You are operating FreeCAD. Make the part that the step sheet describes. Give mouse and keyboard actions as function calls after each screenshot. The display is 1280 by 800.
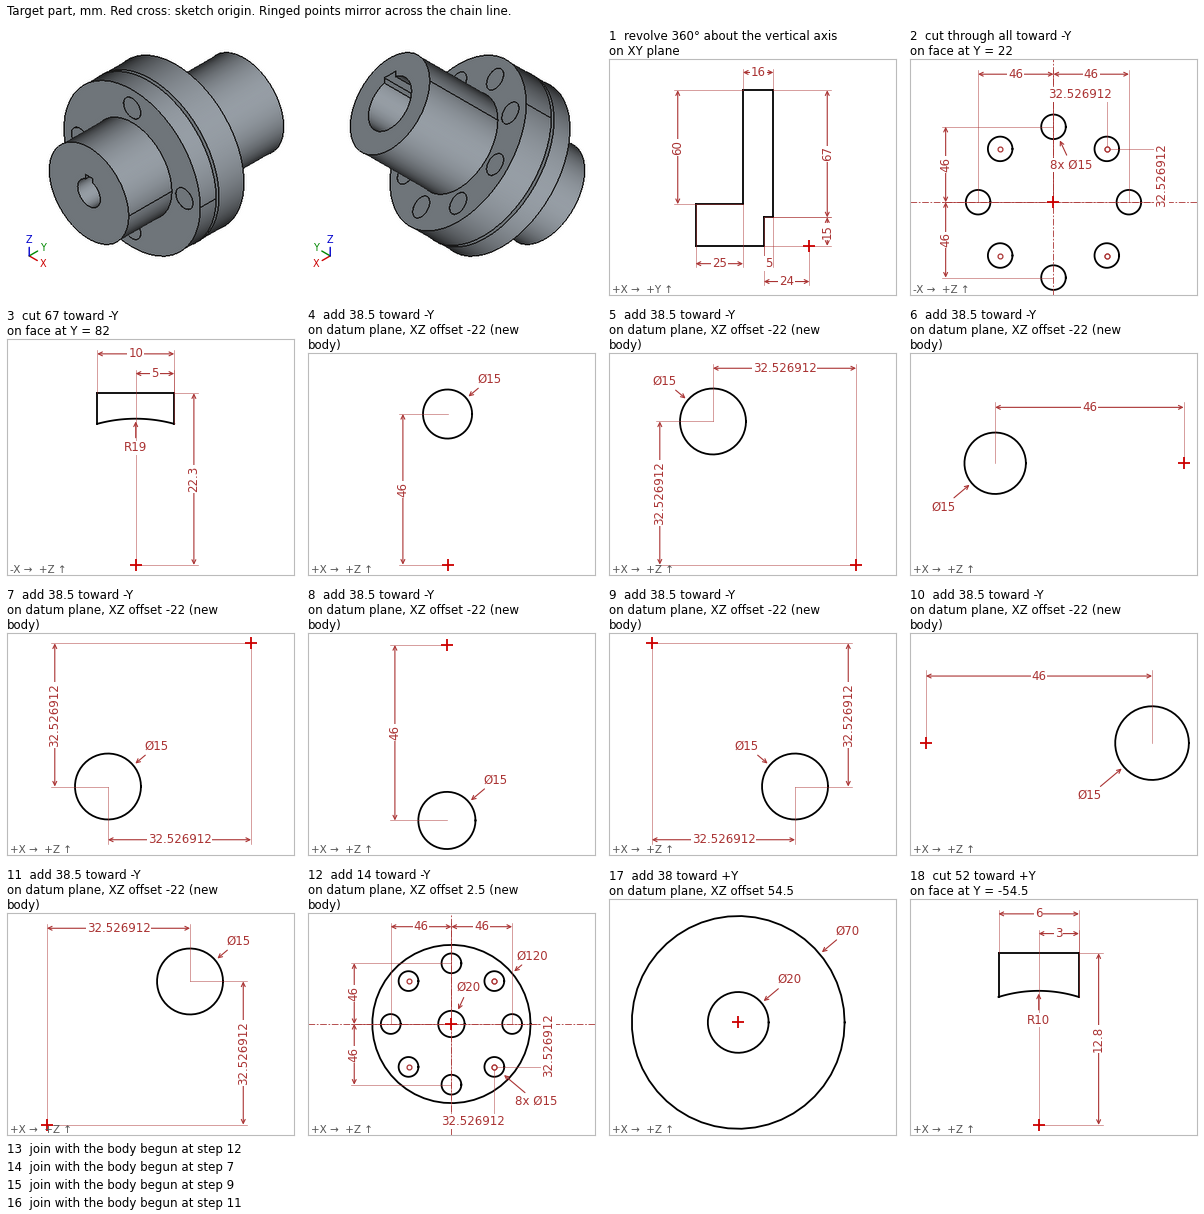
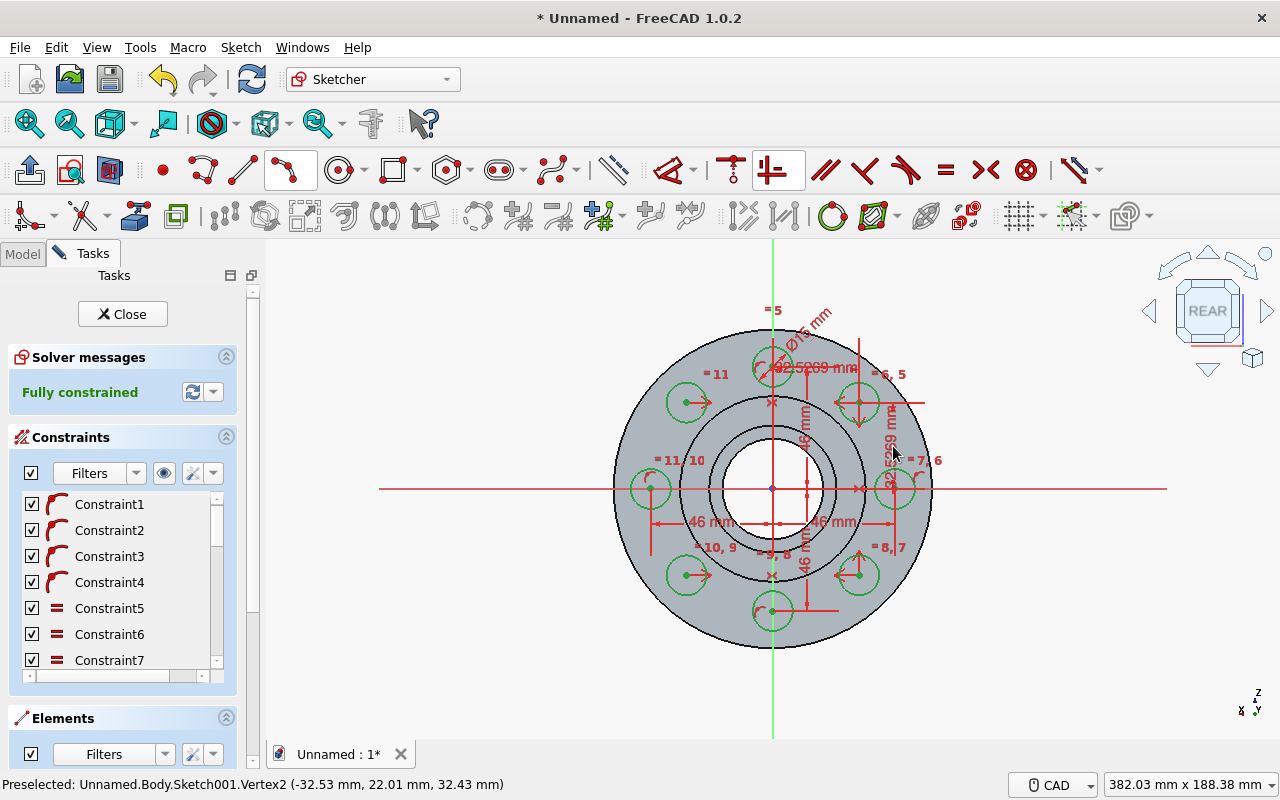
click(123, 314)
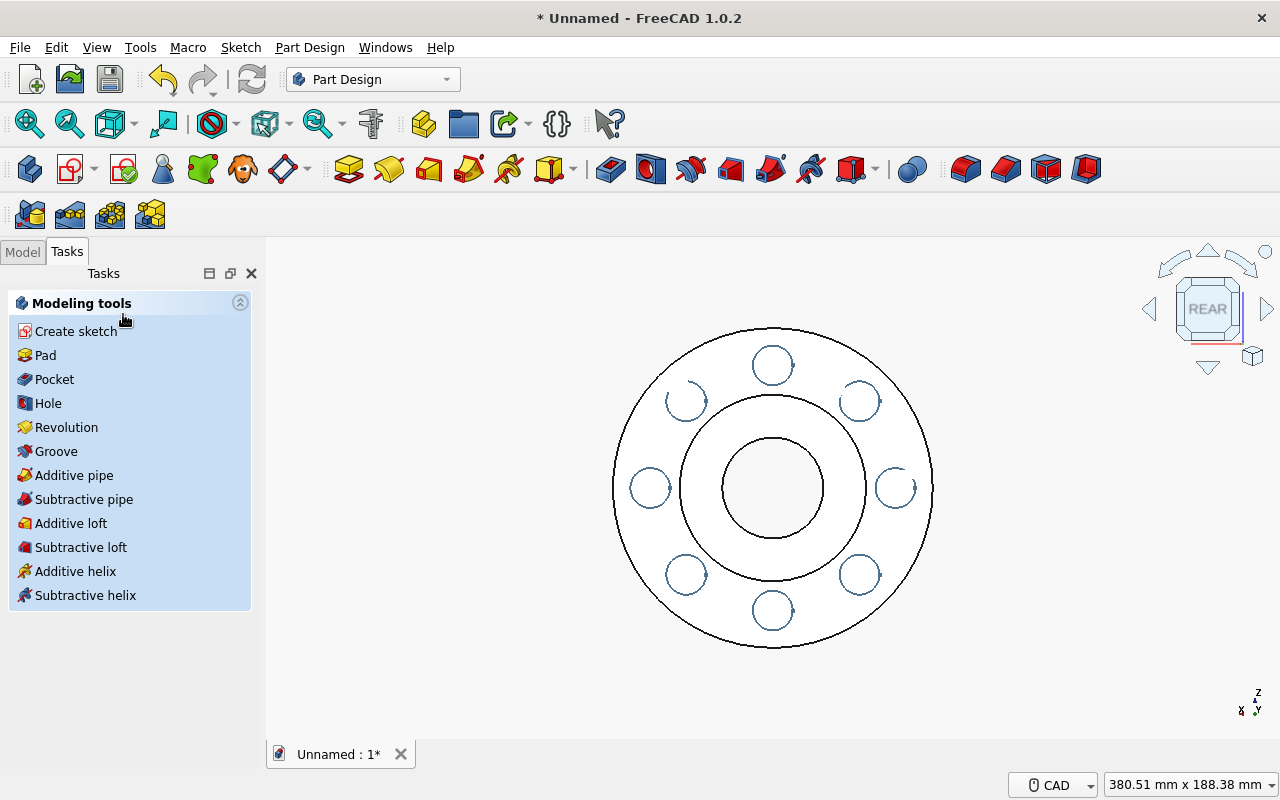
click(612, 170)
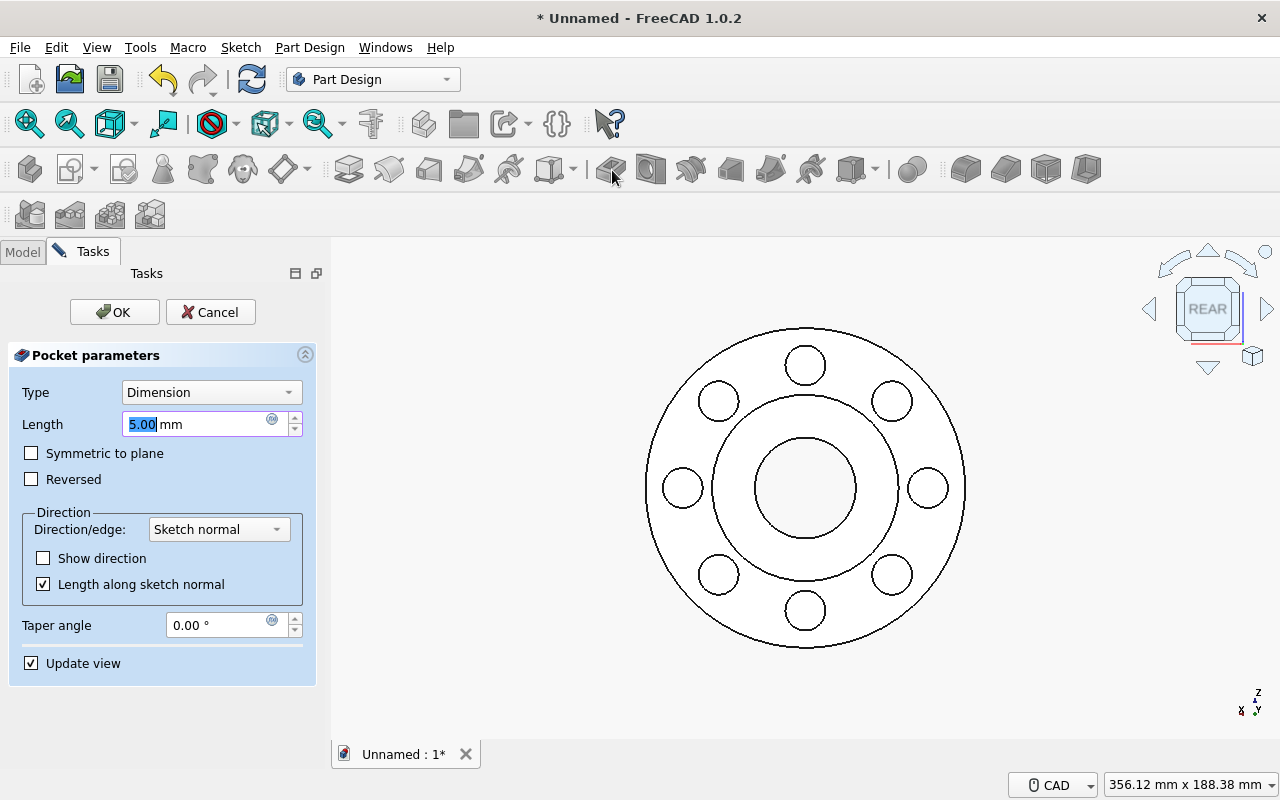
click(212, 392)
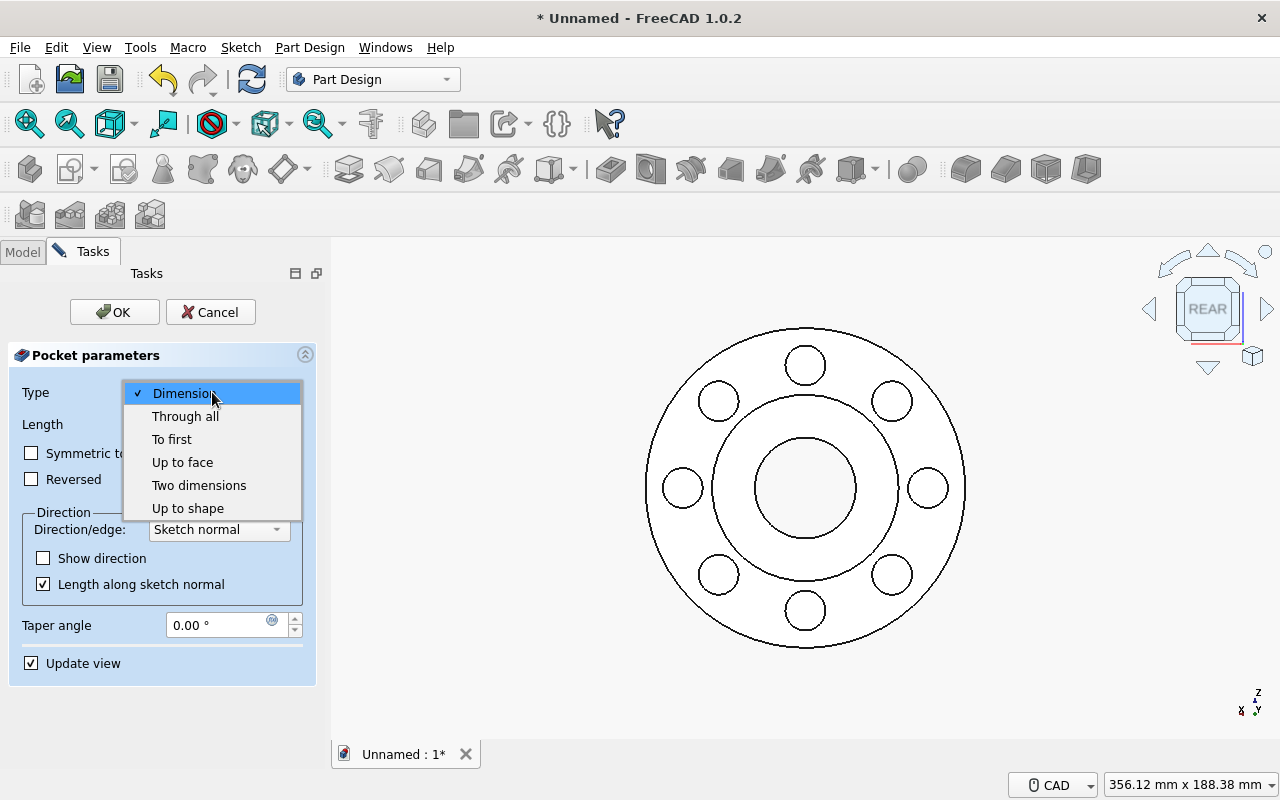
click(212, 416)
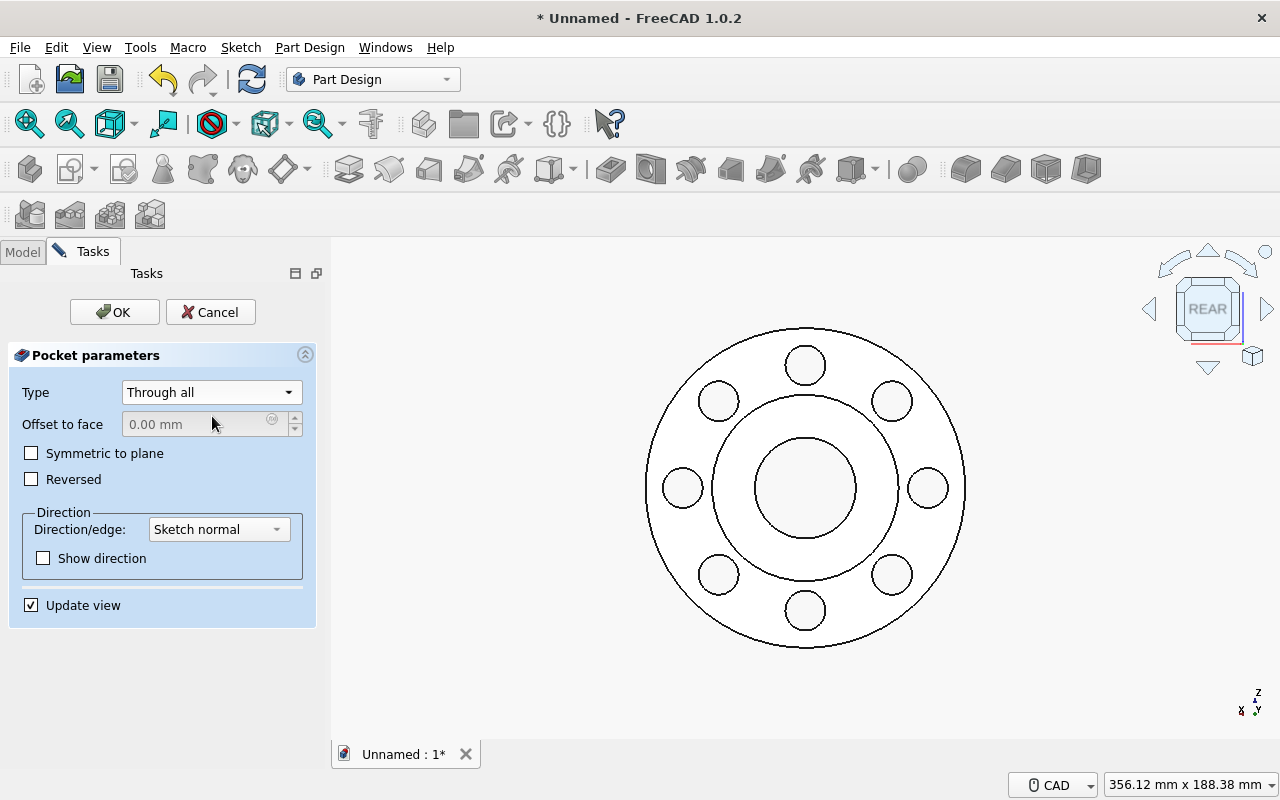
click(115, 312)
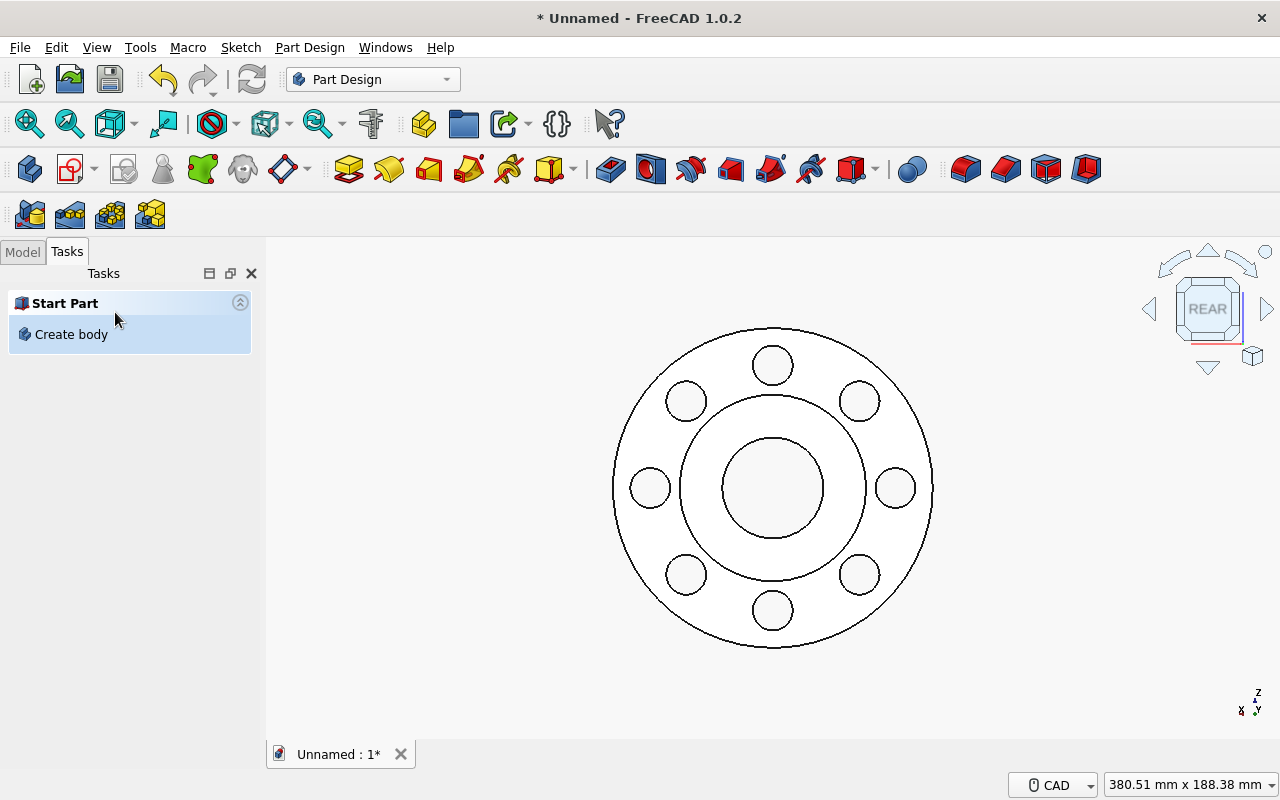
click(720, 540)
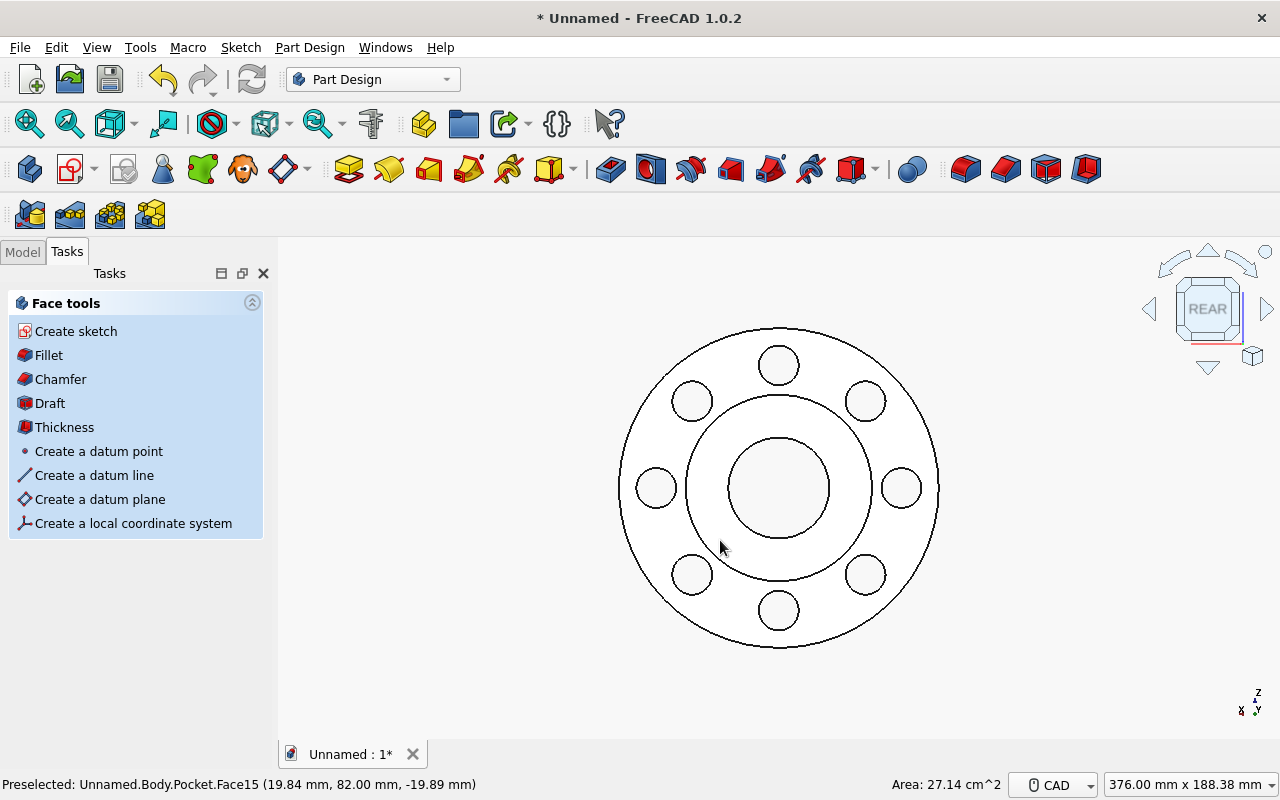
click(70, 170)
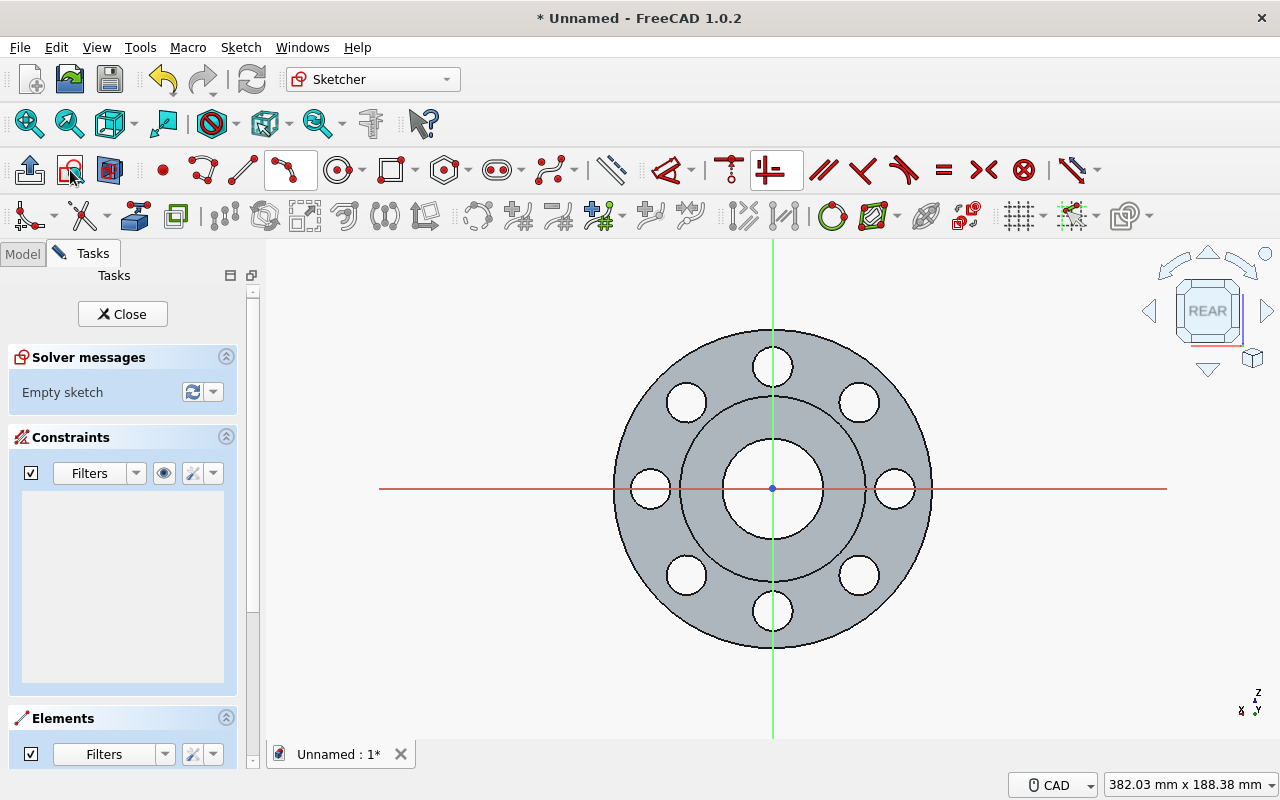
scroll(790, 452, up, 8)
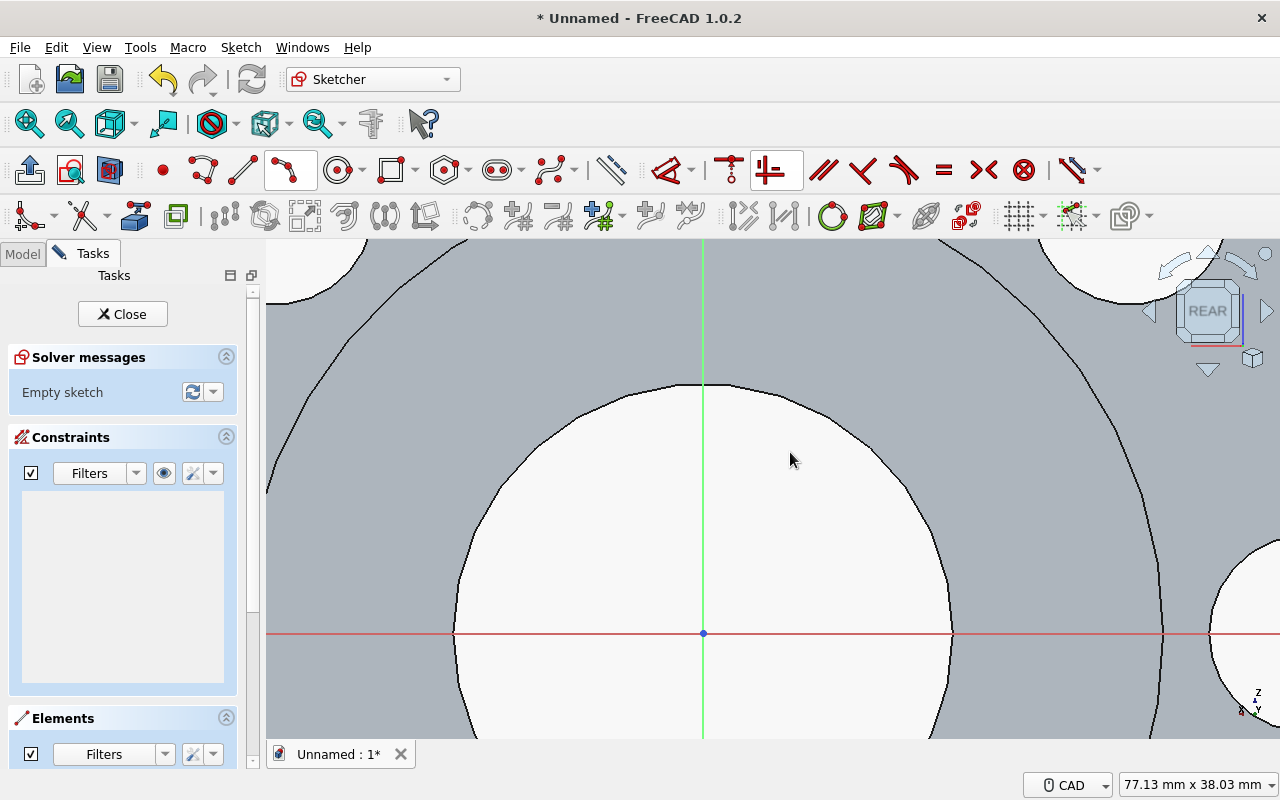
click(204, 170)